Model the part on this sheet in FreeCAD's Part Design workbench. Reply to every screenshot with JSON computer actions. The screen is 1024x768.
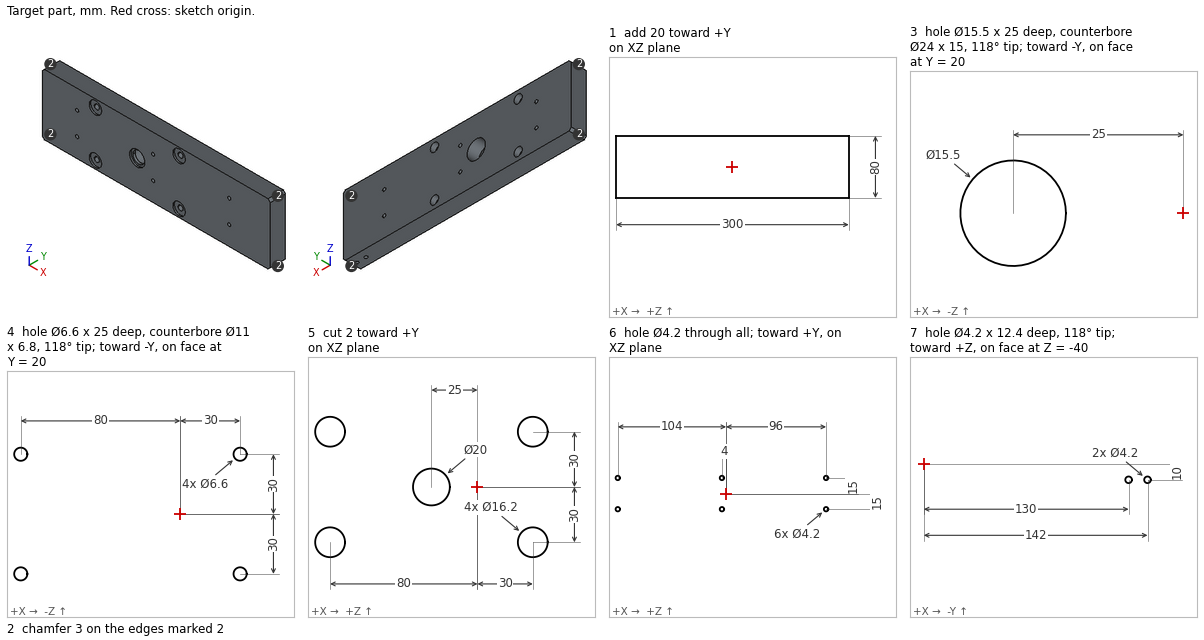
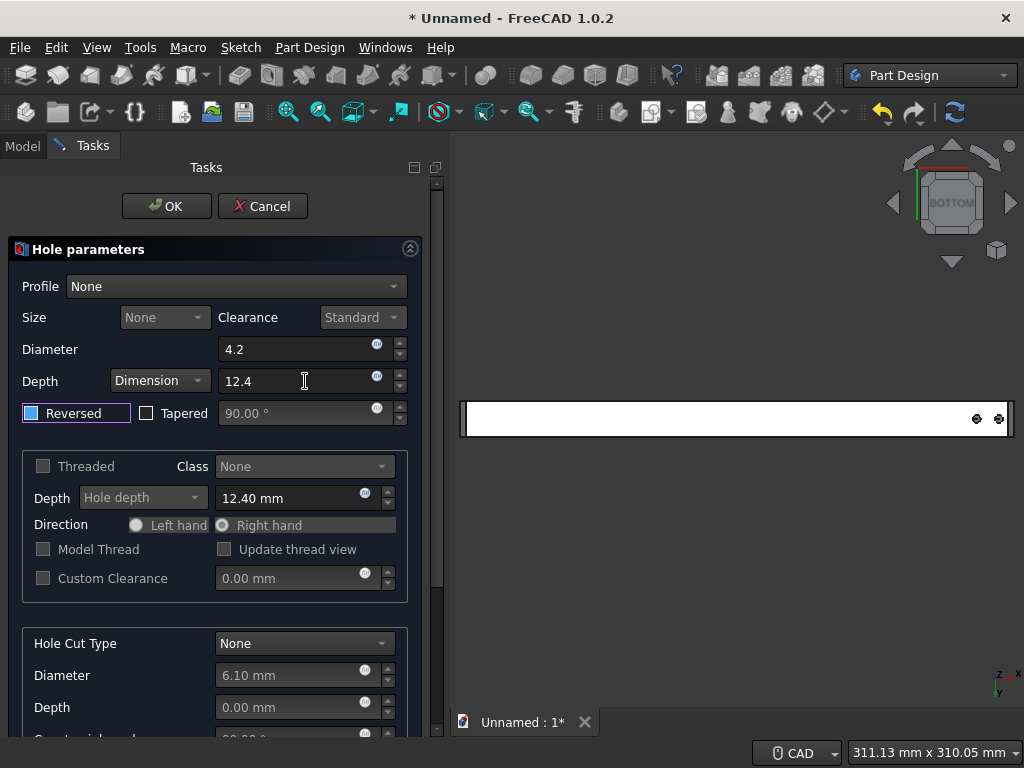
{"action": "left_click", "coordinate": [167, 206]}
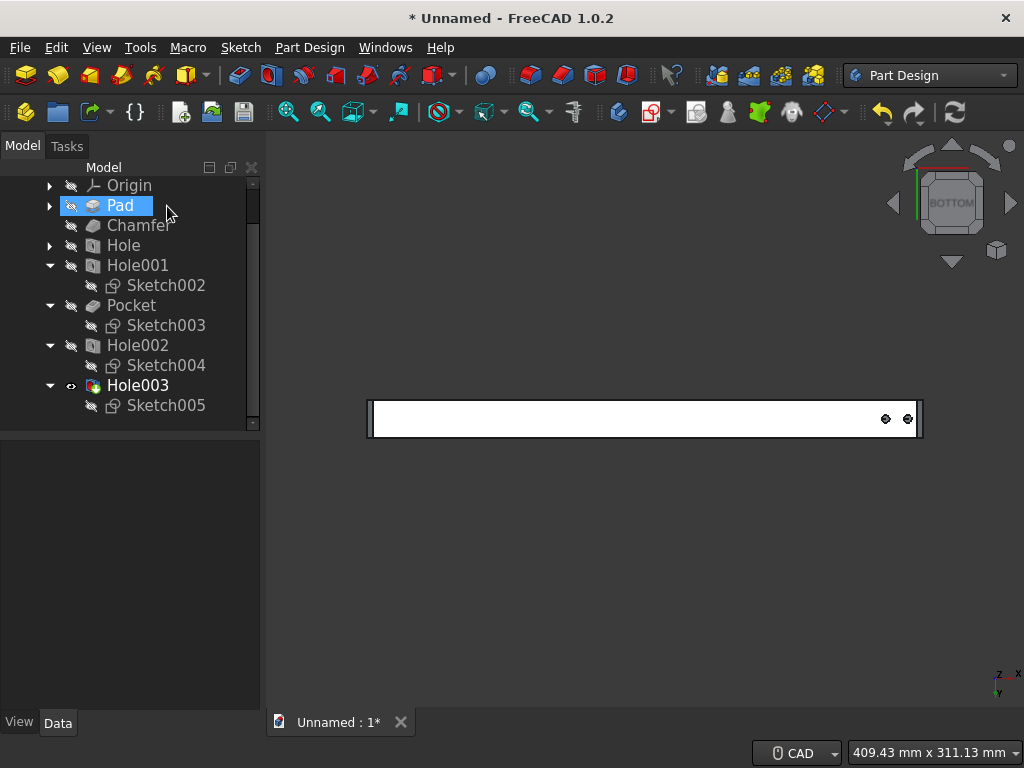
{"action": "key", "text": "0"}